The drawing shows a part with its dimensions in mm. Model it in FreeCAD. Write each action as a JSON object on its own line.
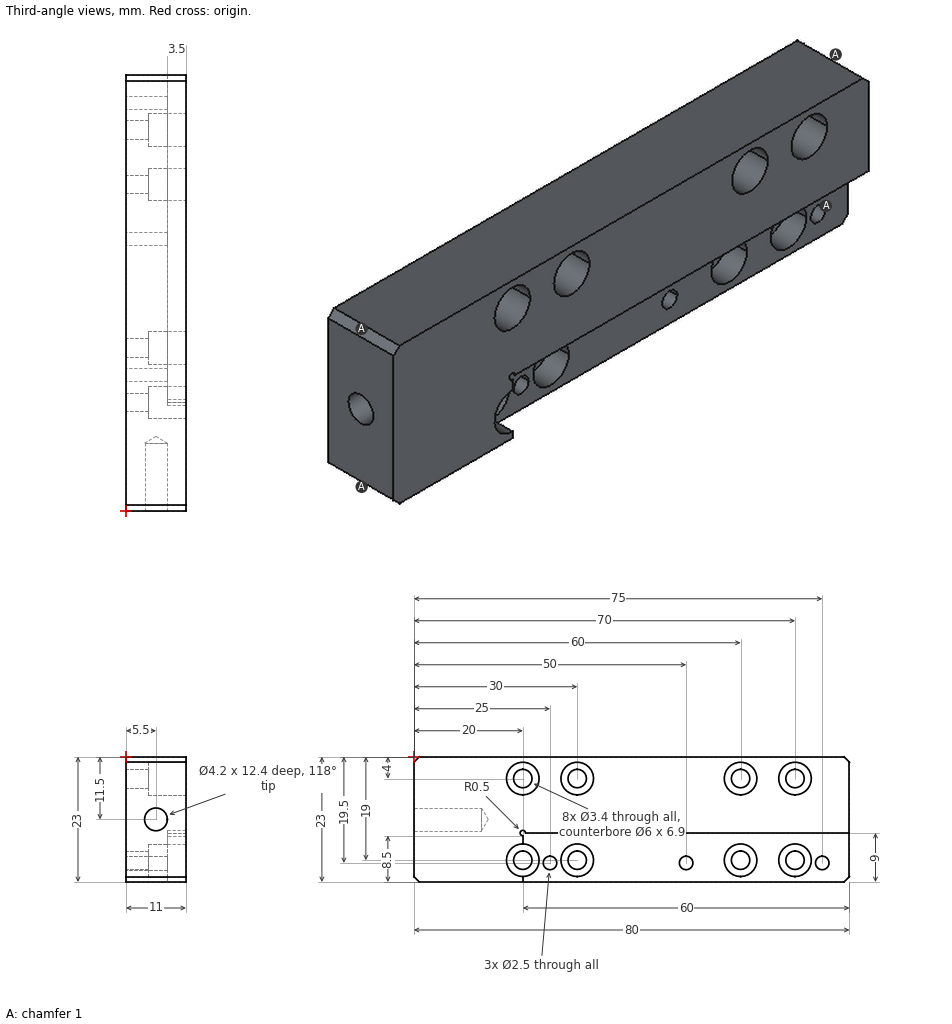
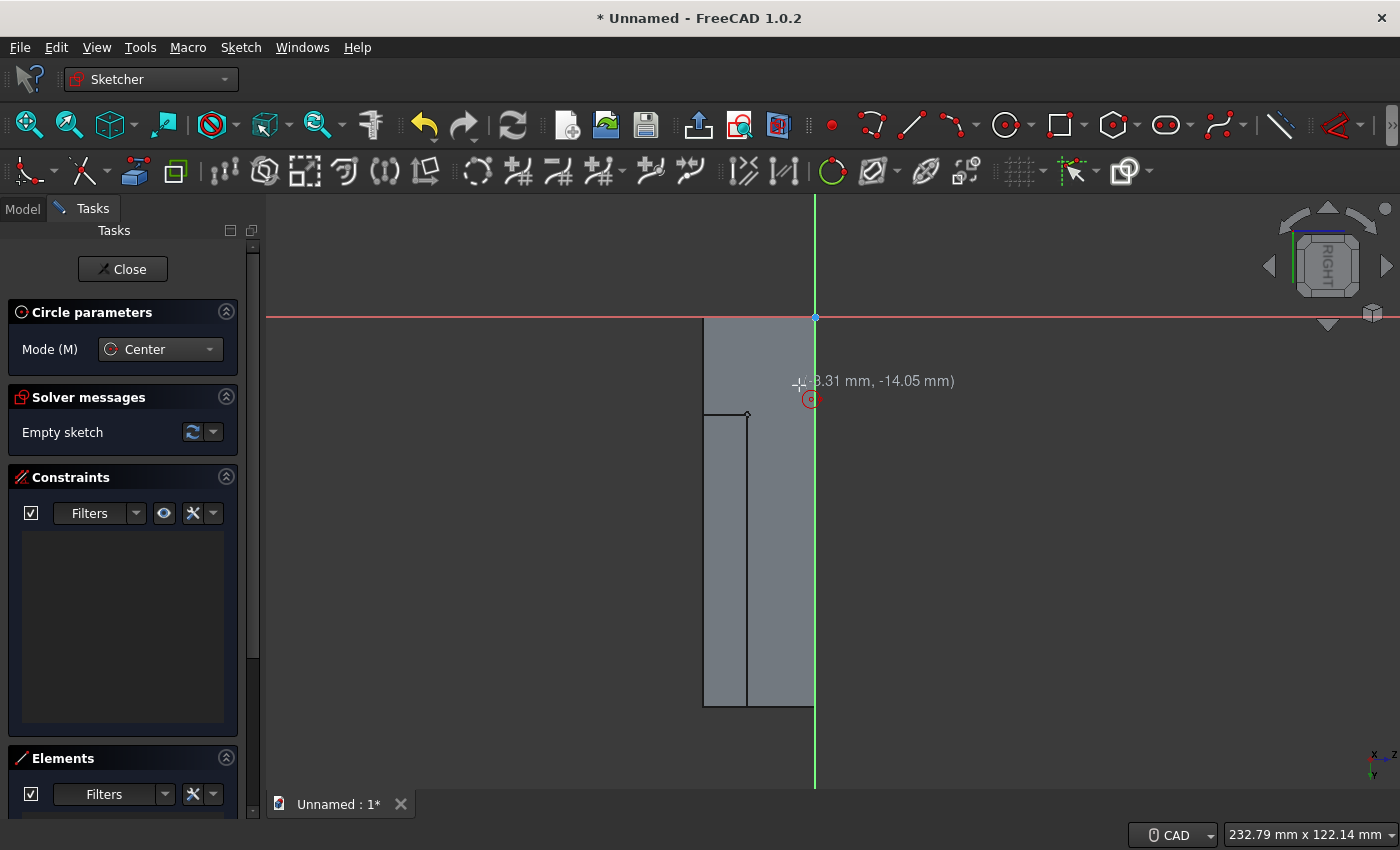
{"action": "left_click", "coordinate": [796, 415]}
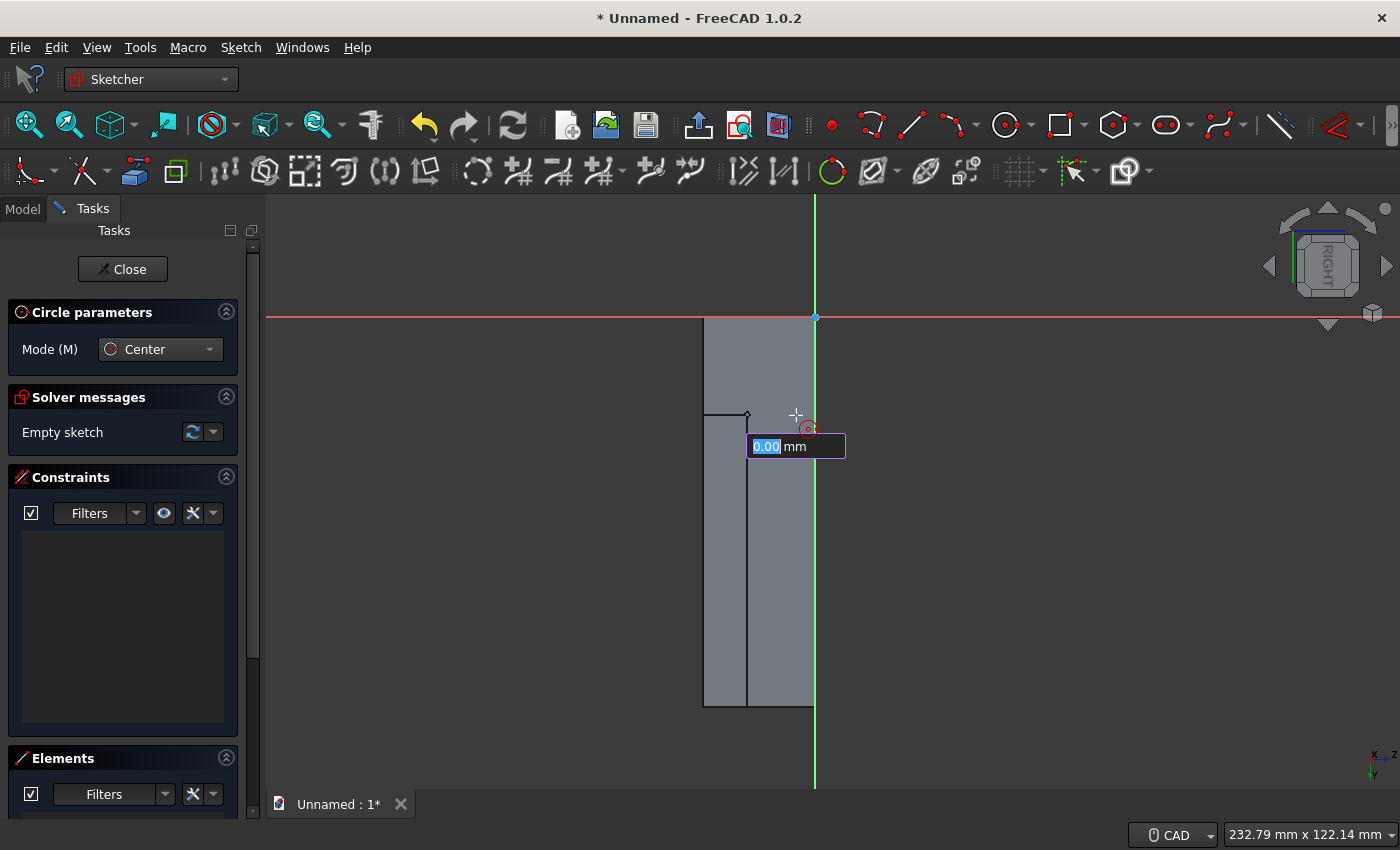
{"action": "scroll", "coordinate": [790, 409], "scroll_direction": "up", "scroll_amount": 4}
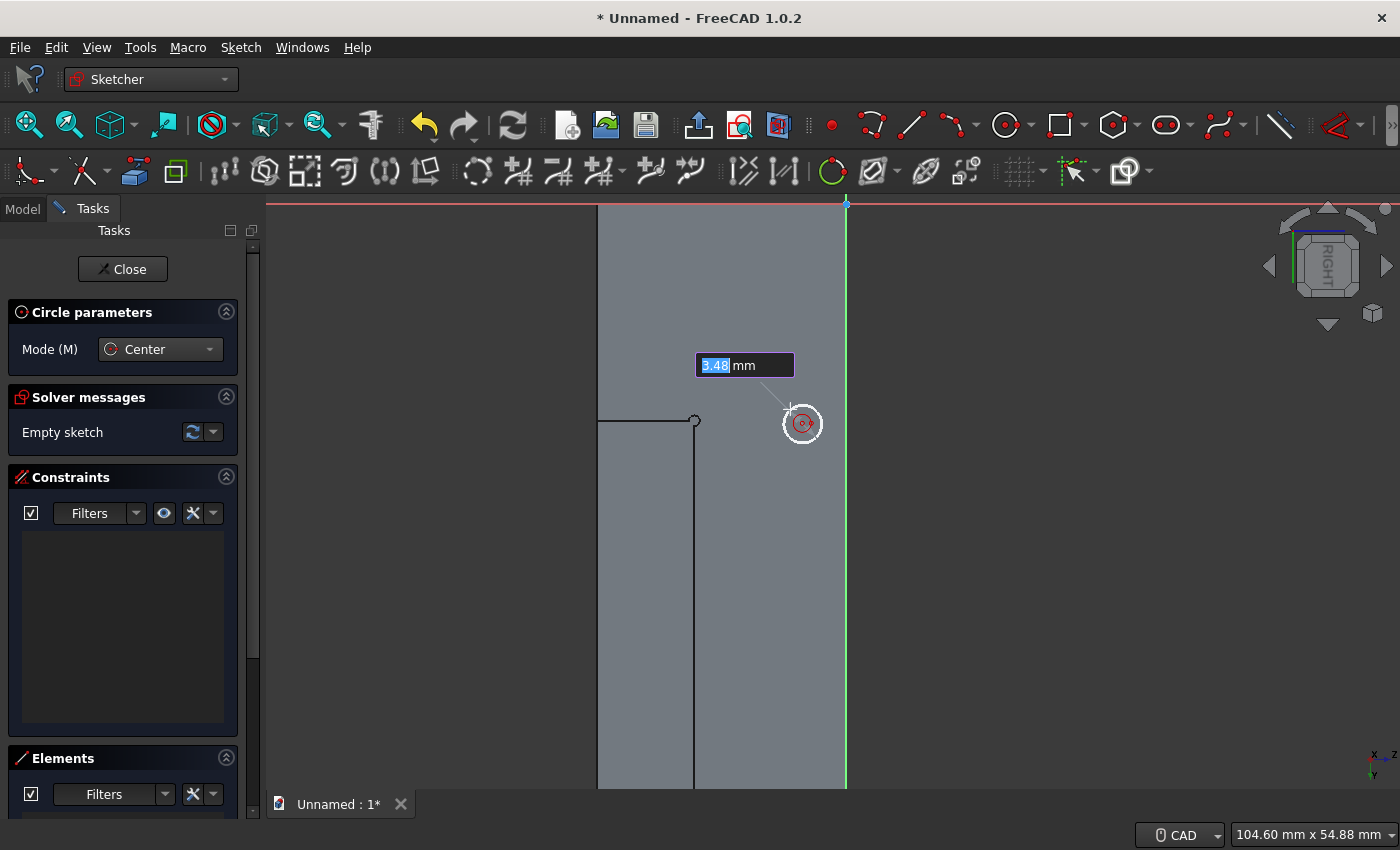
{"action": "left_click", "coordinate": [790, 408]}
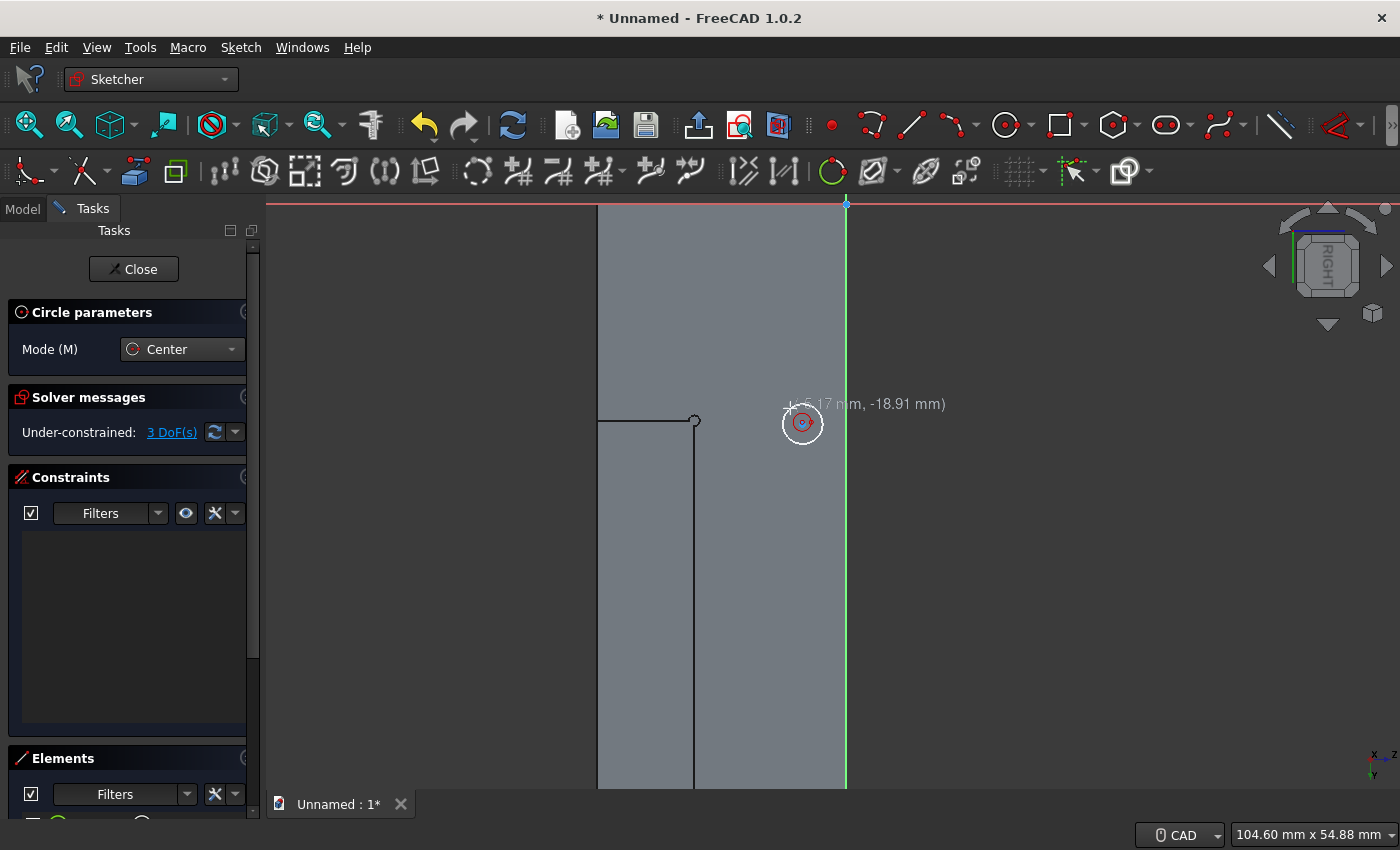
{"action": "scroll", "coordinate": [803, 529], "scroll_direction": "up", "scroll_amount": 2}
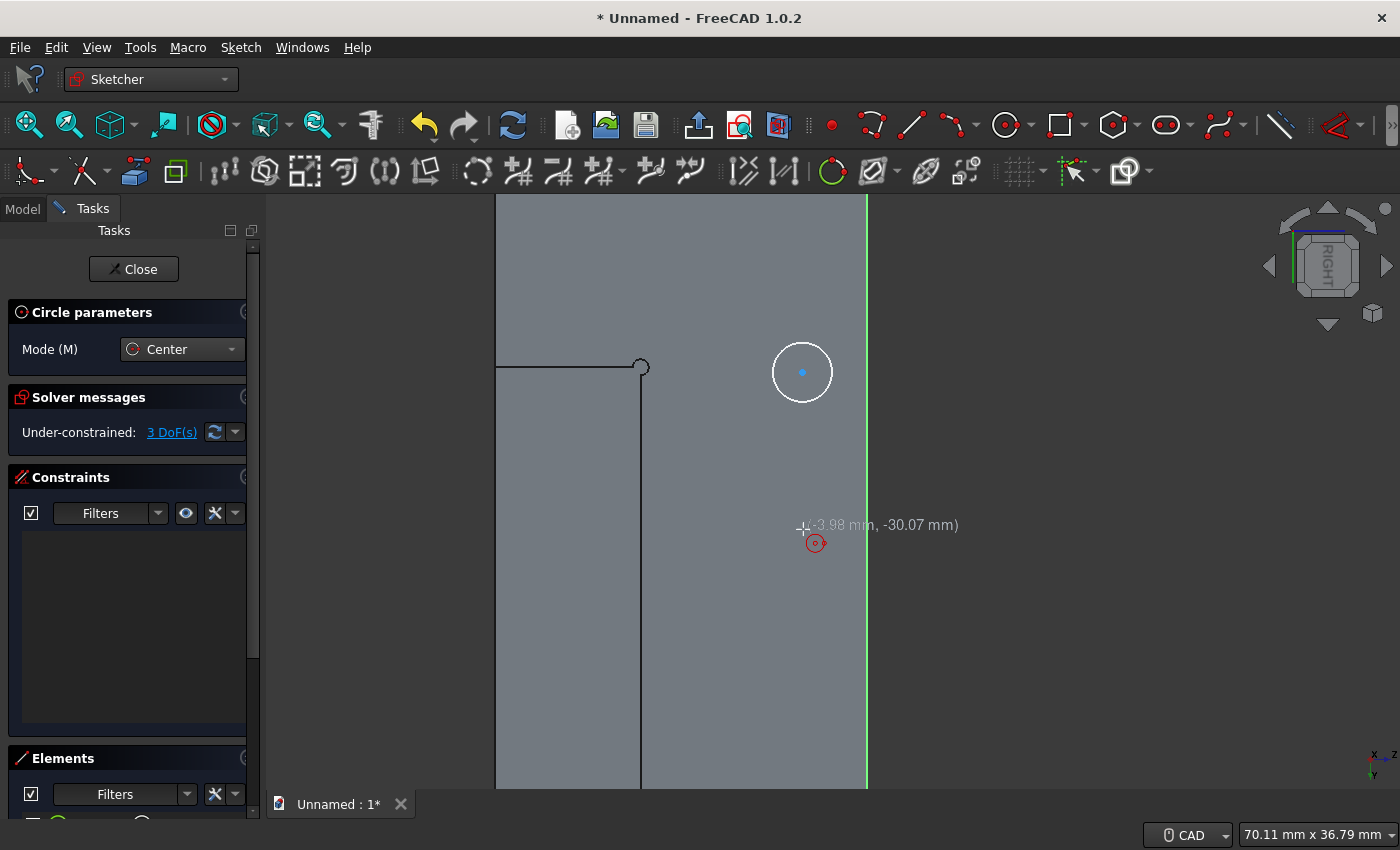
{"action": "scroll", "coordinate": [792, 435], "scroll_direction": "down", "scroll_amount": 6}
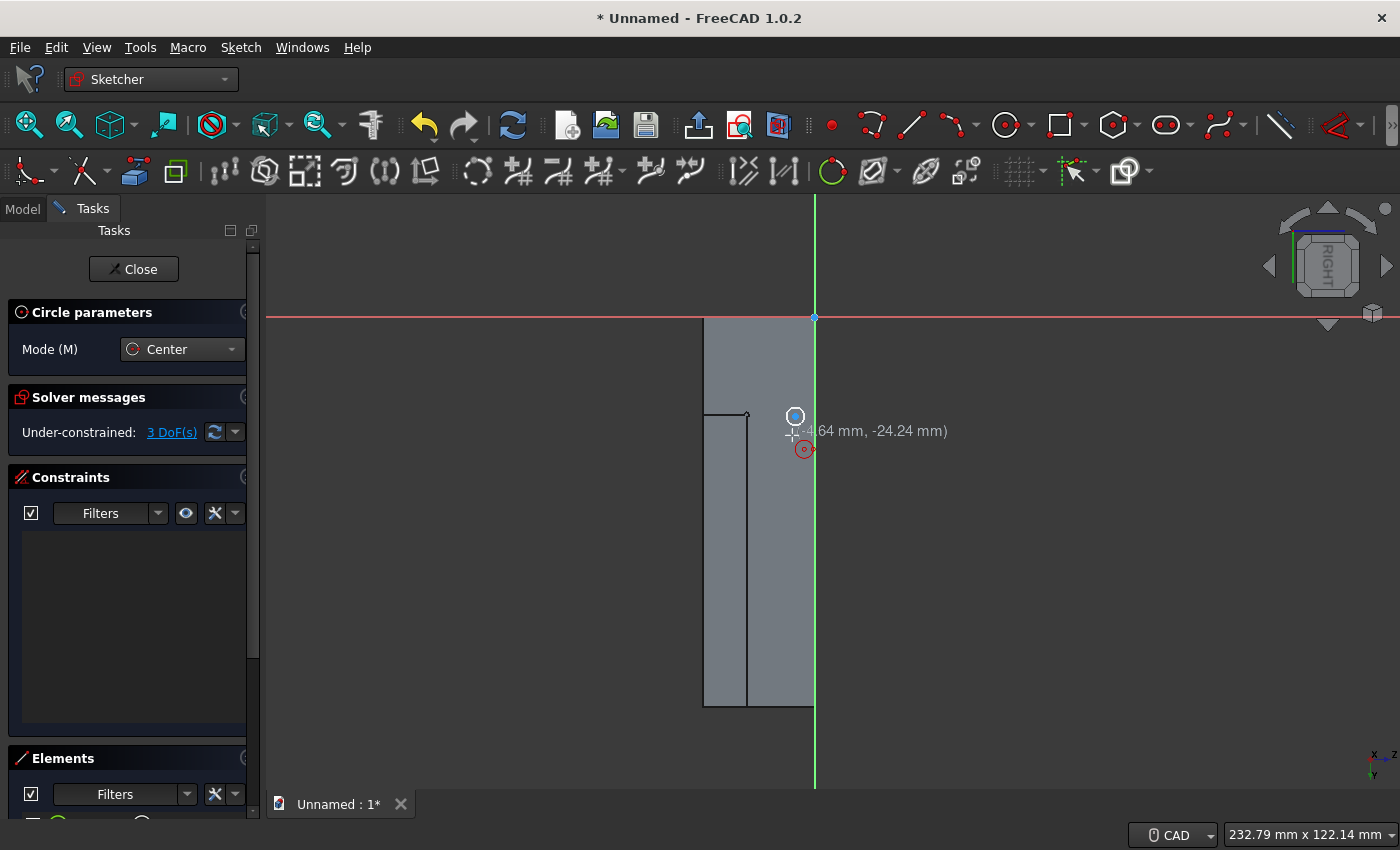
{"action": "left_click", "coordinate": [795, 464]}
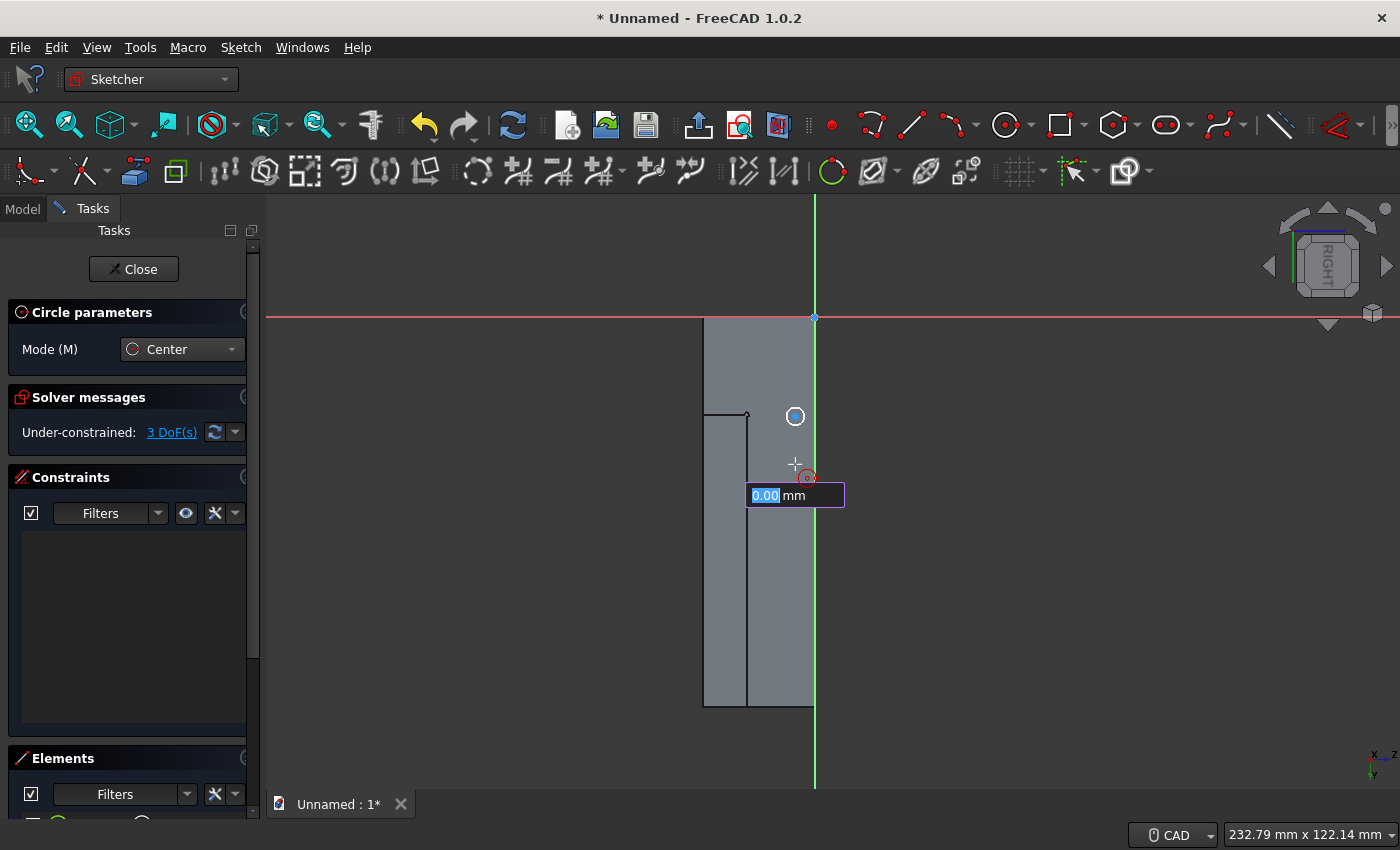
{"action": "scroll", "coordinate": [790, 458], "scroll_direction": "up", "scroll_amount": 4}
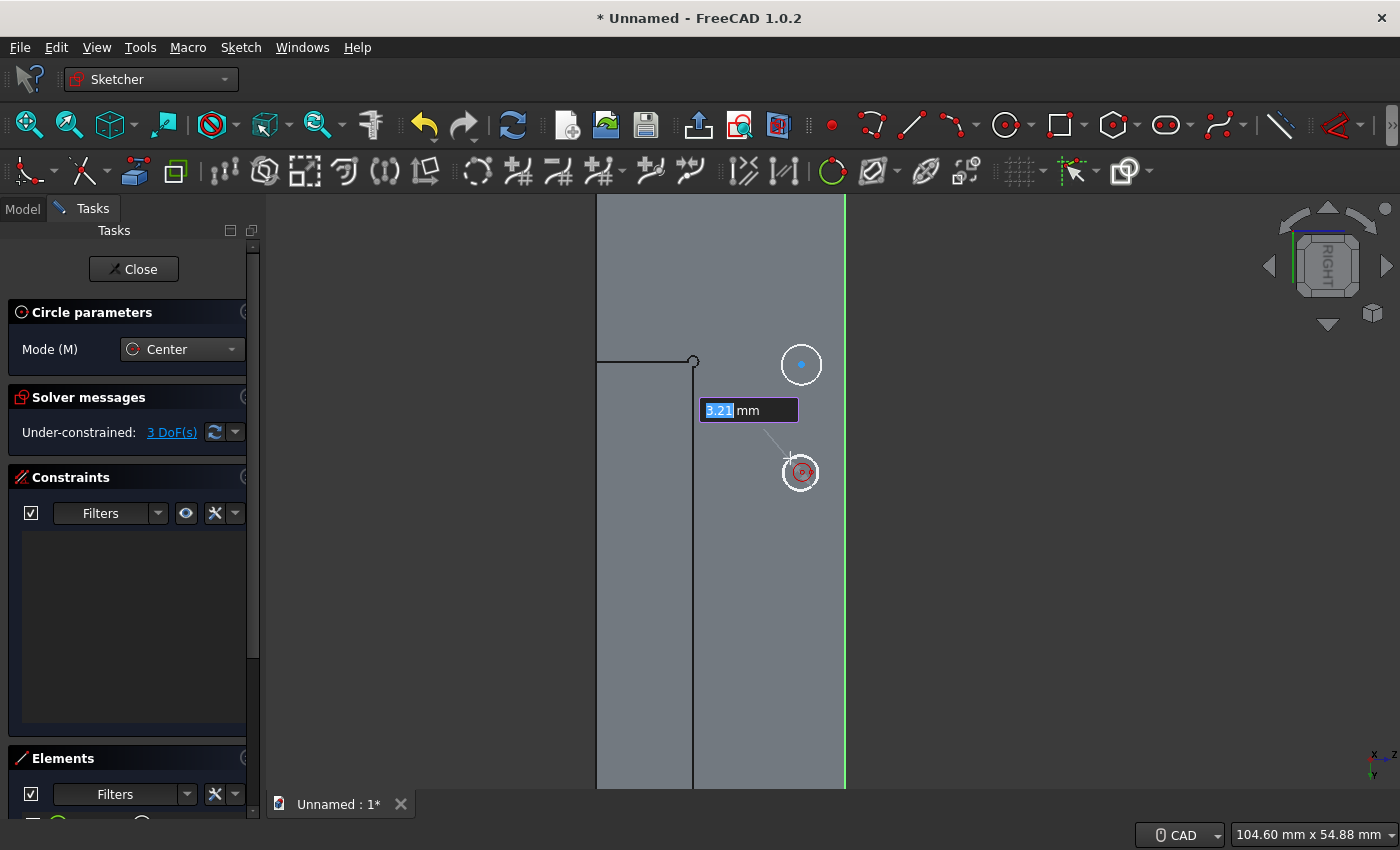
{"action": "left_click", "coordinate": [789, 457]}